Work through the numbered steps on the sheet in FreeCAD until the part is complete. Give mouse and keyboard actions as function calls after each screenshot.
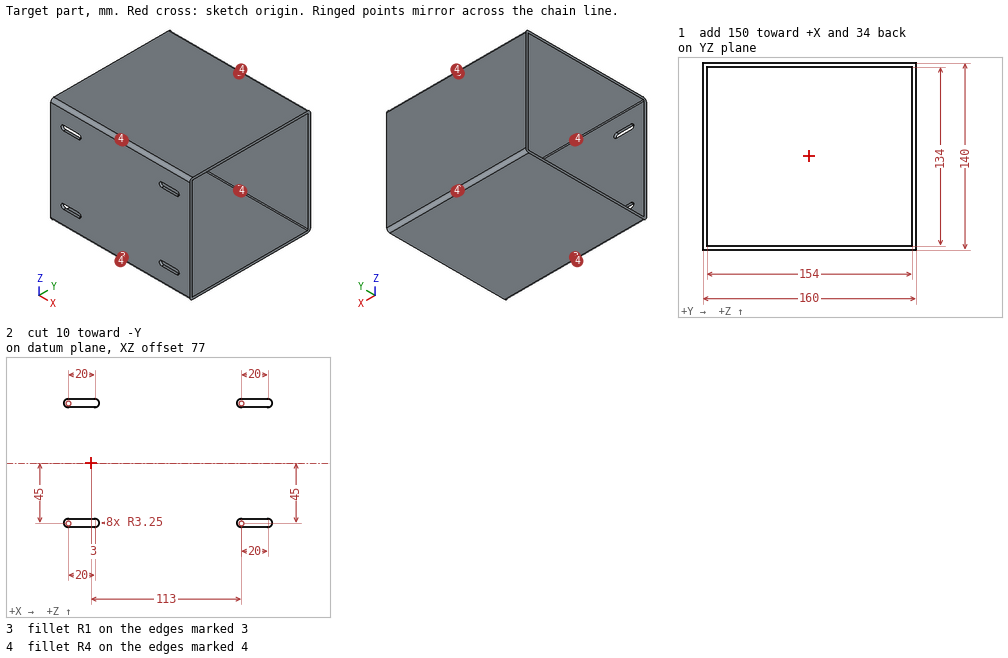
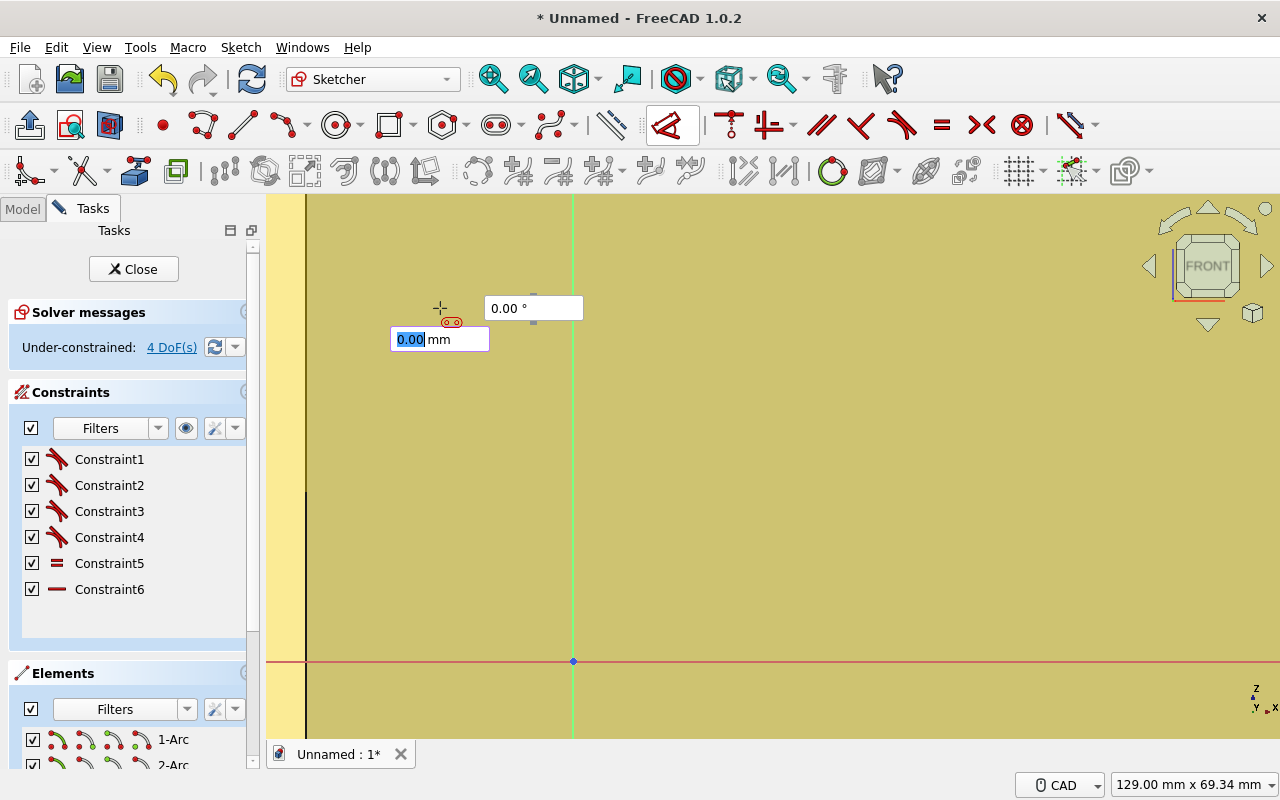
click(597, 308)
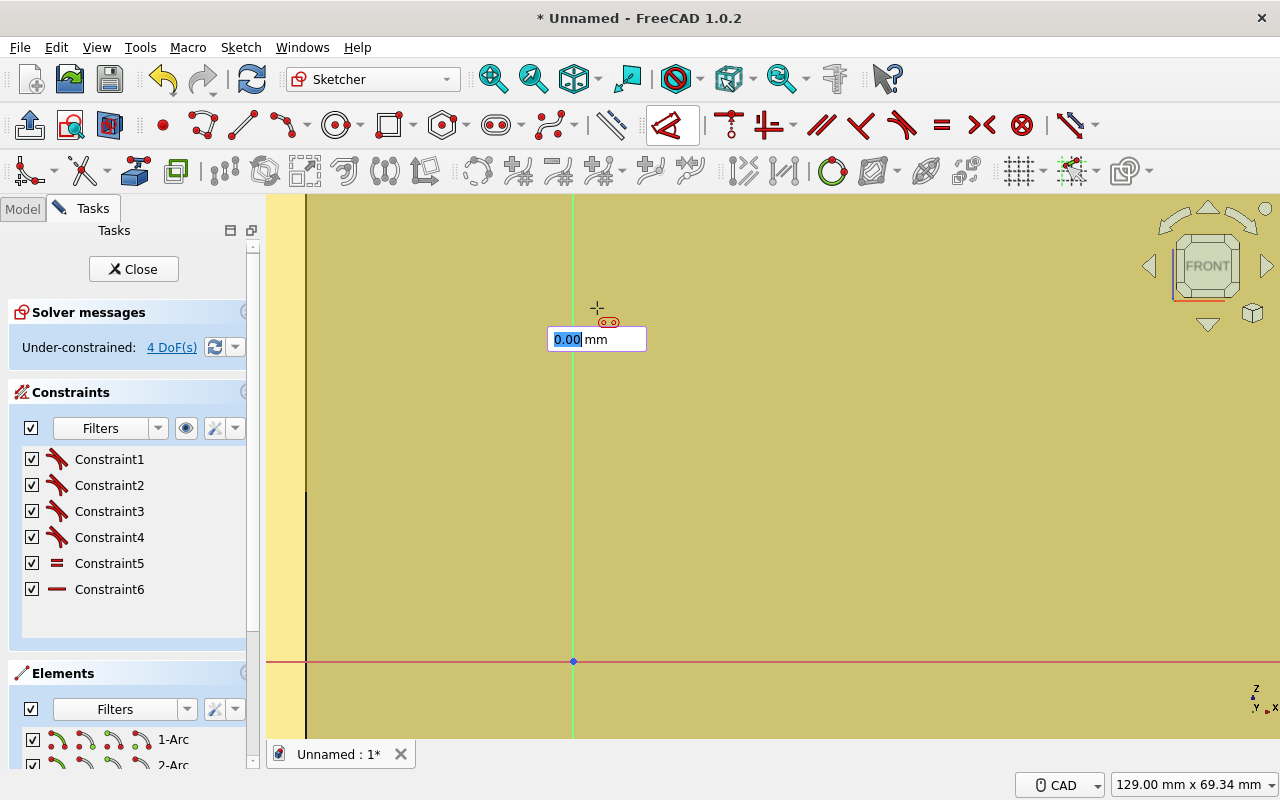
click(518, 282)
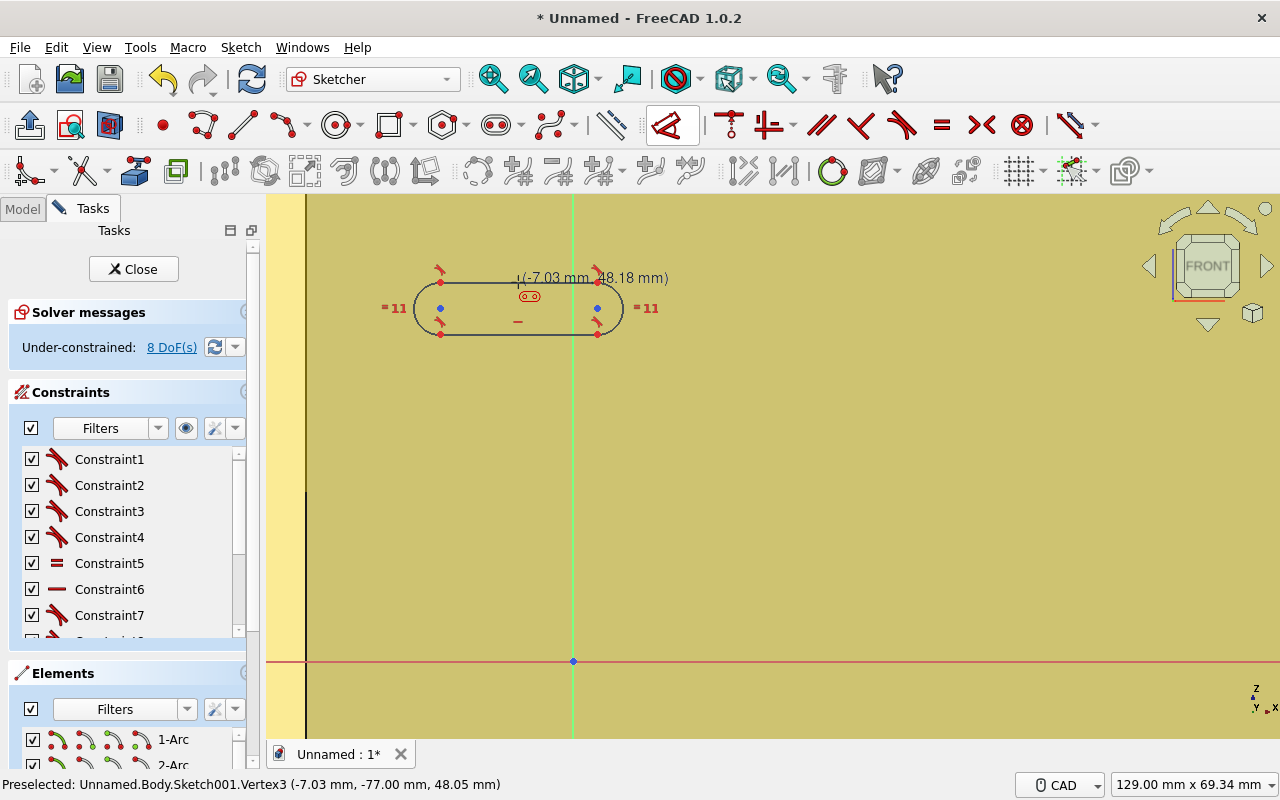
scroll(440, 307, down, 4)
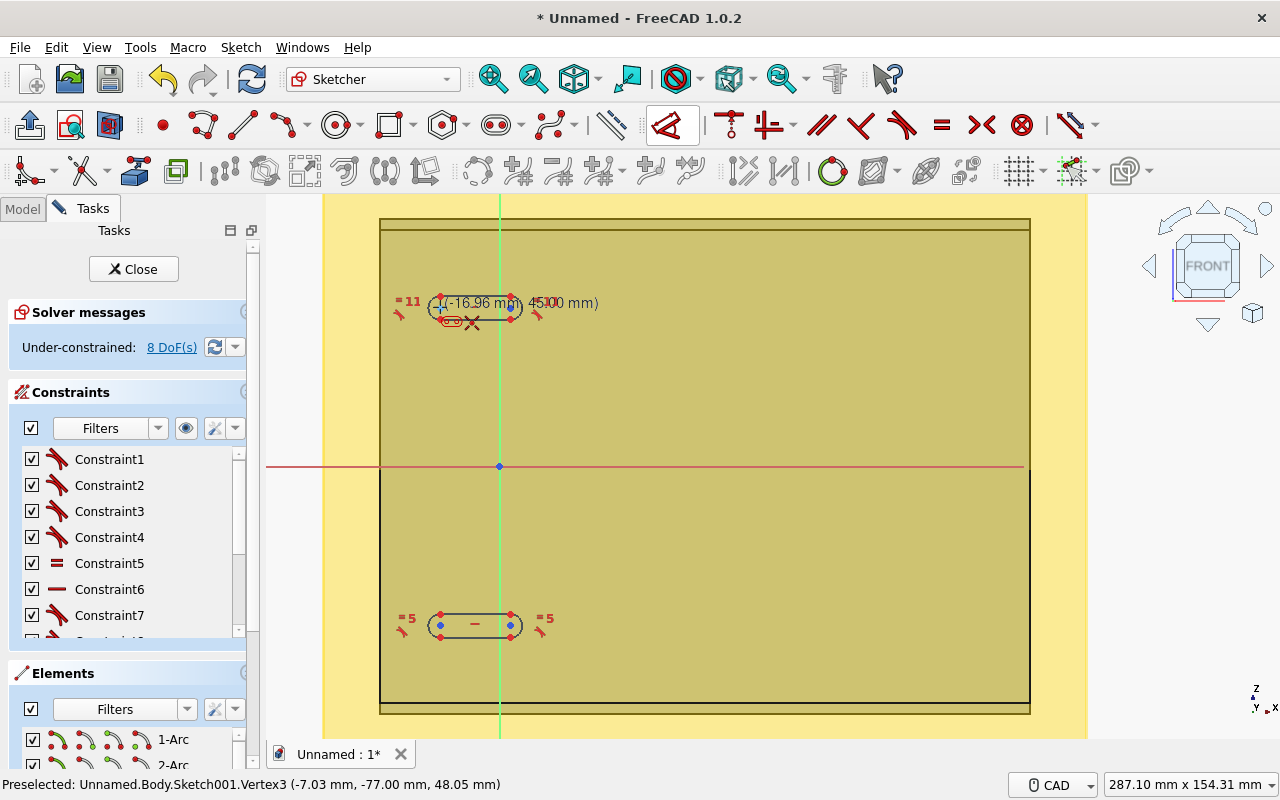
scroll(899, 625, up, 4)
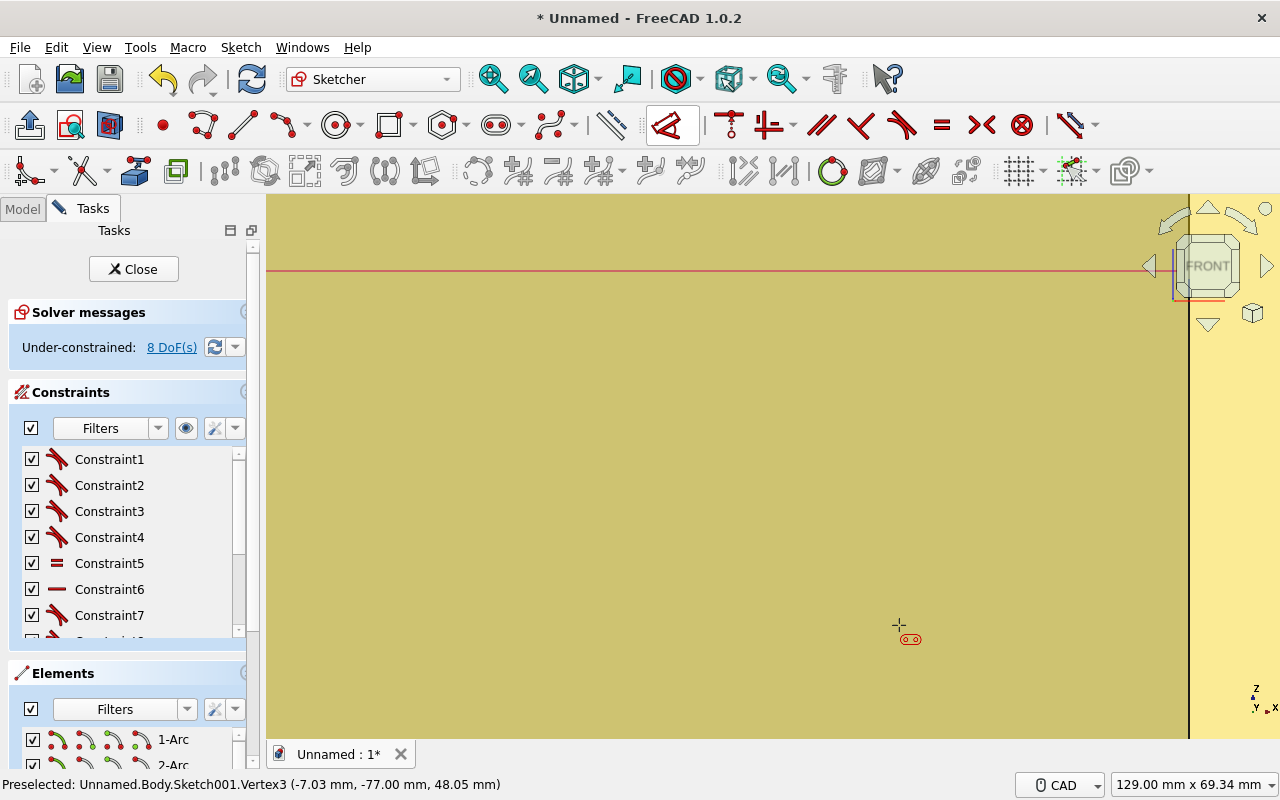
click(898, 625)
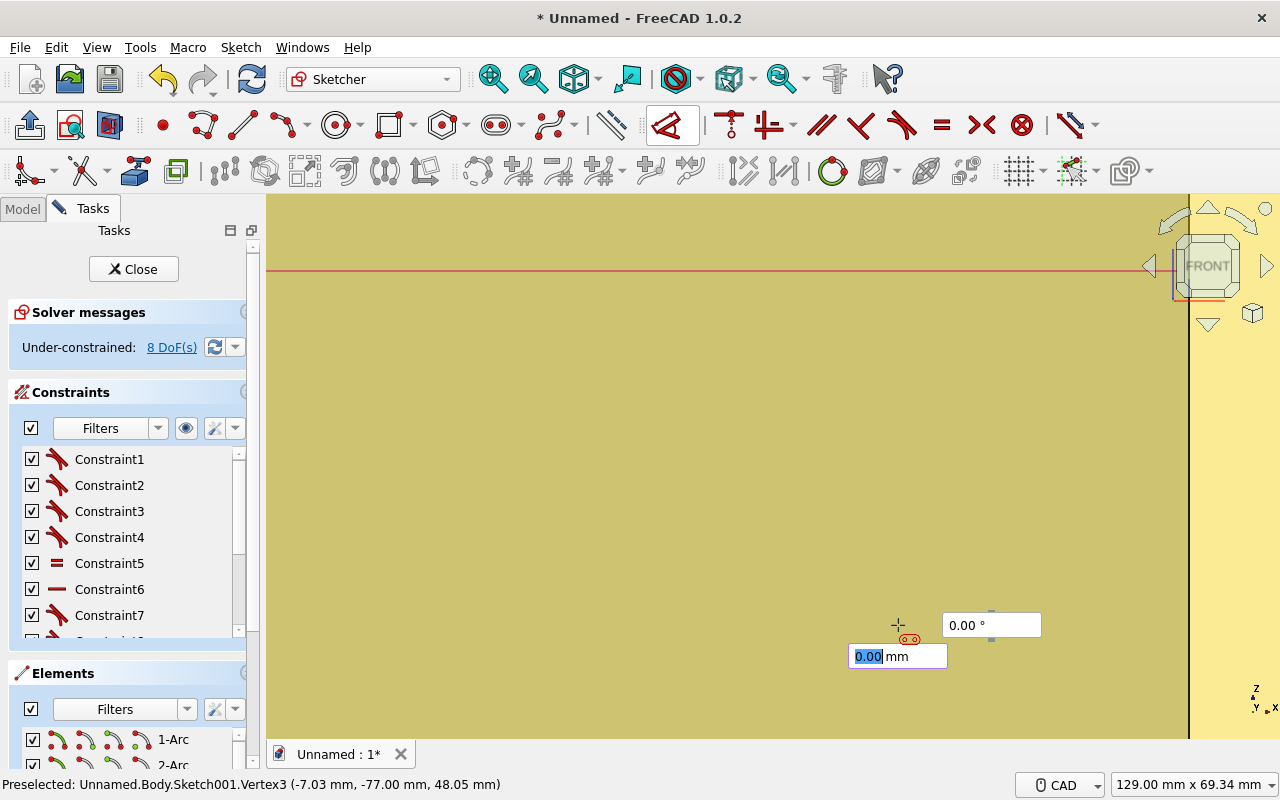
click(1056, 625)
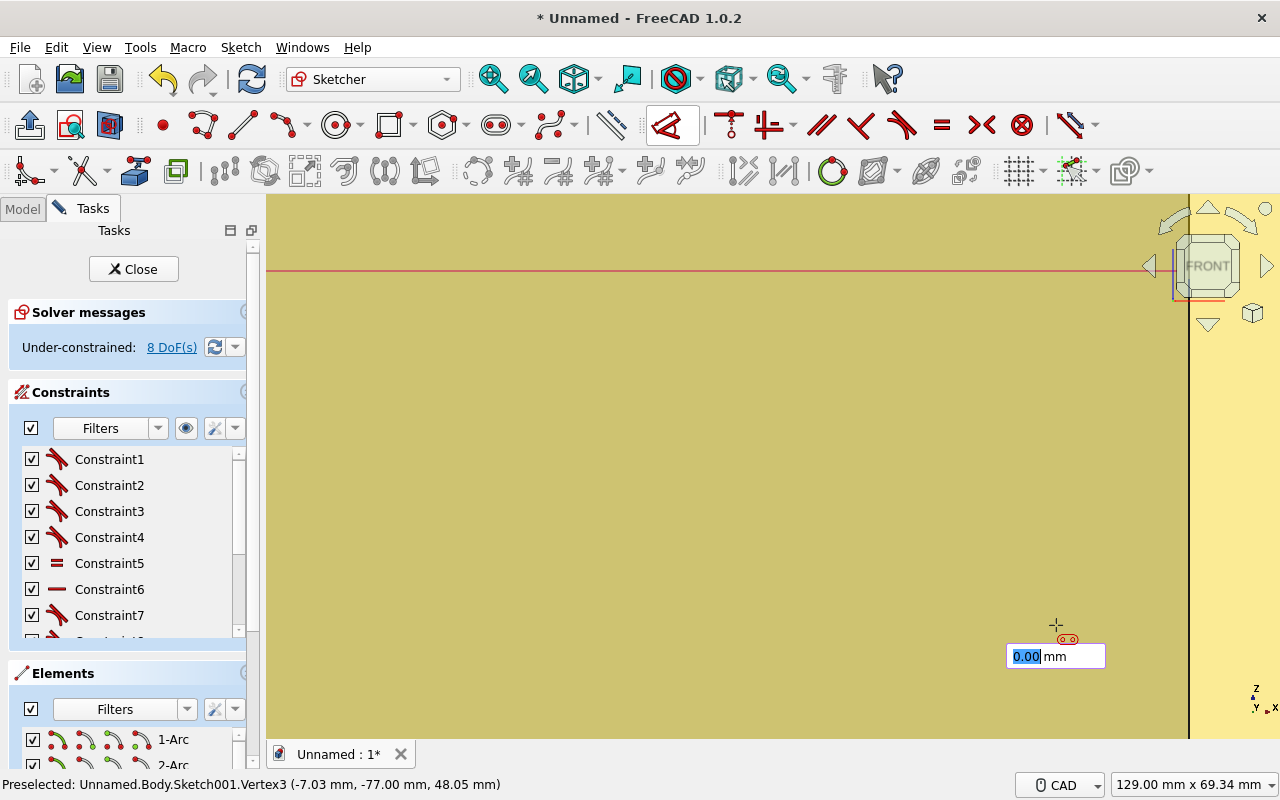
click(977, 651)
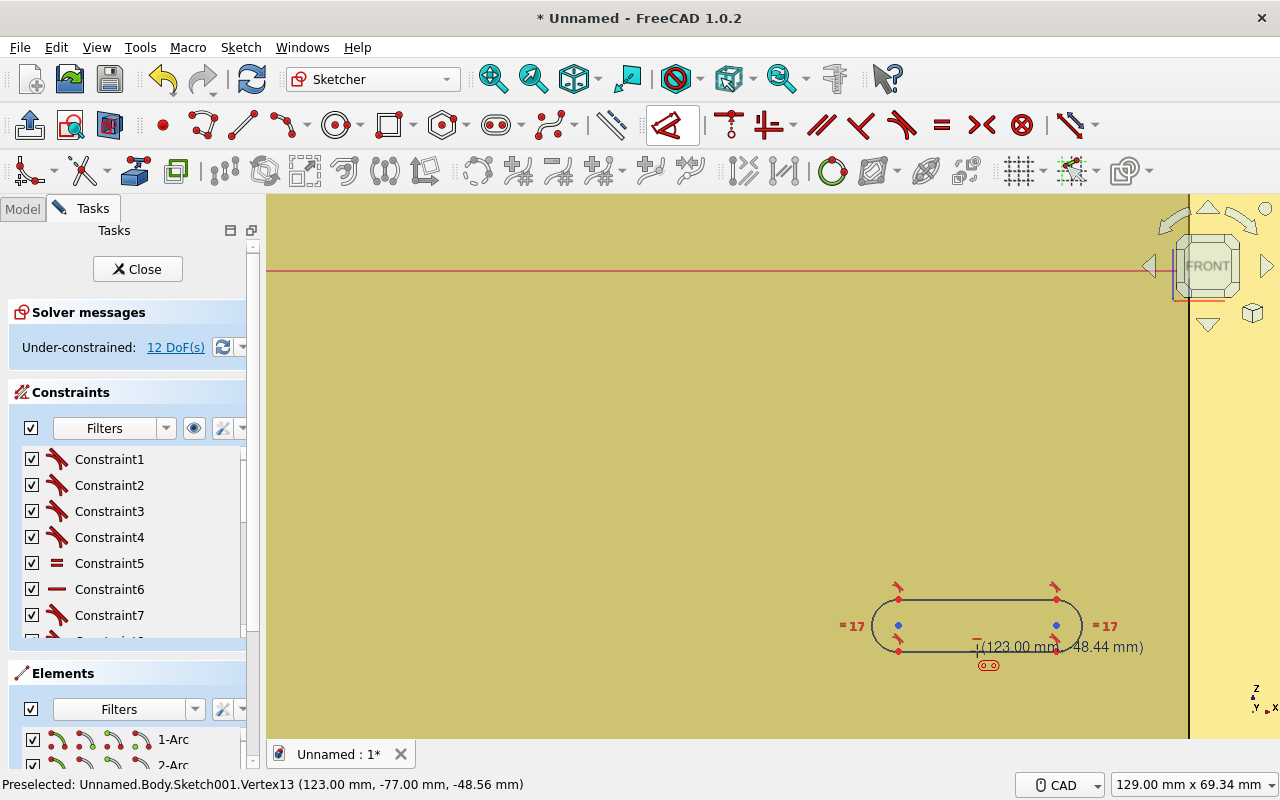
scroll(899, 626, down, 4)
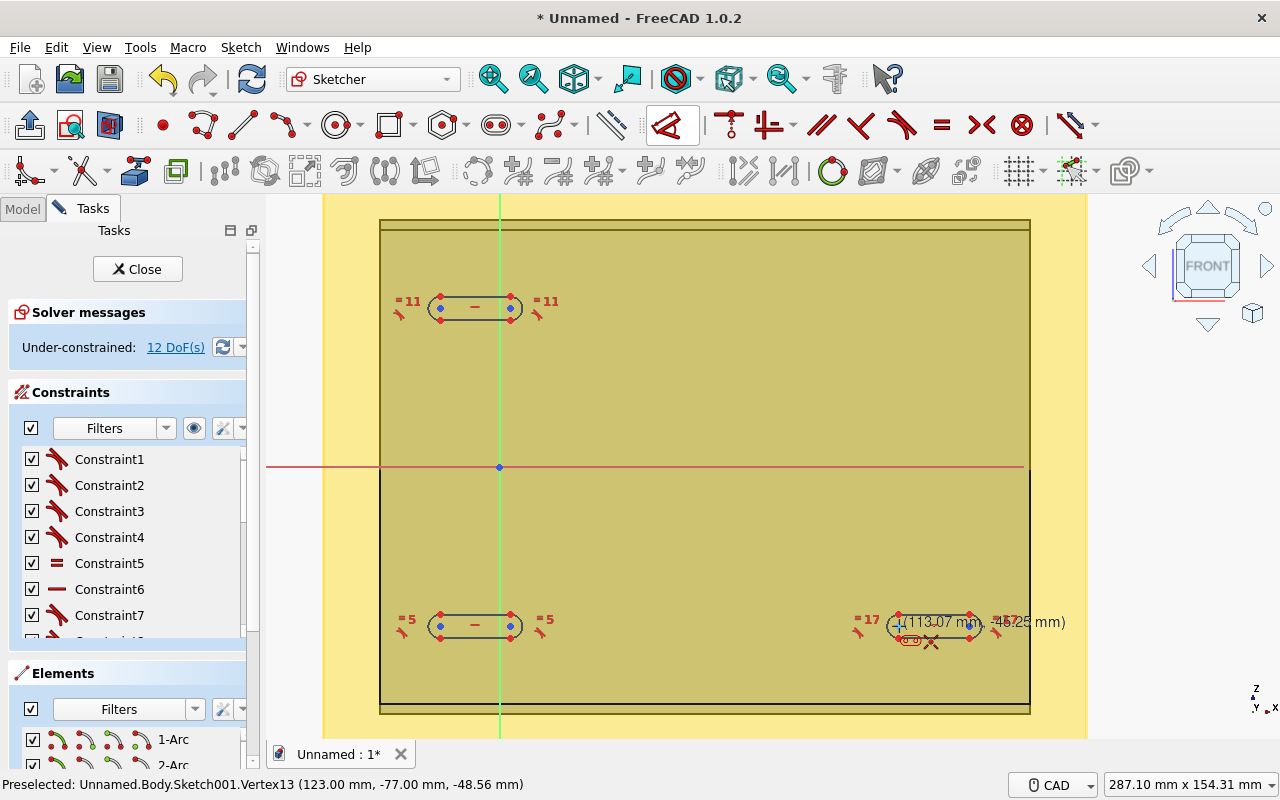
scroll(899, 308, up, 4)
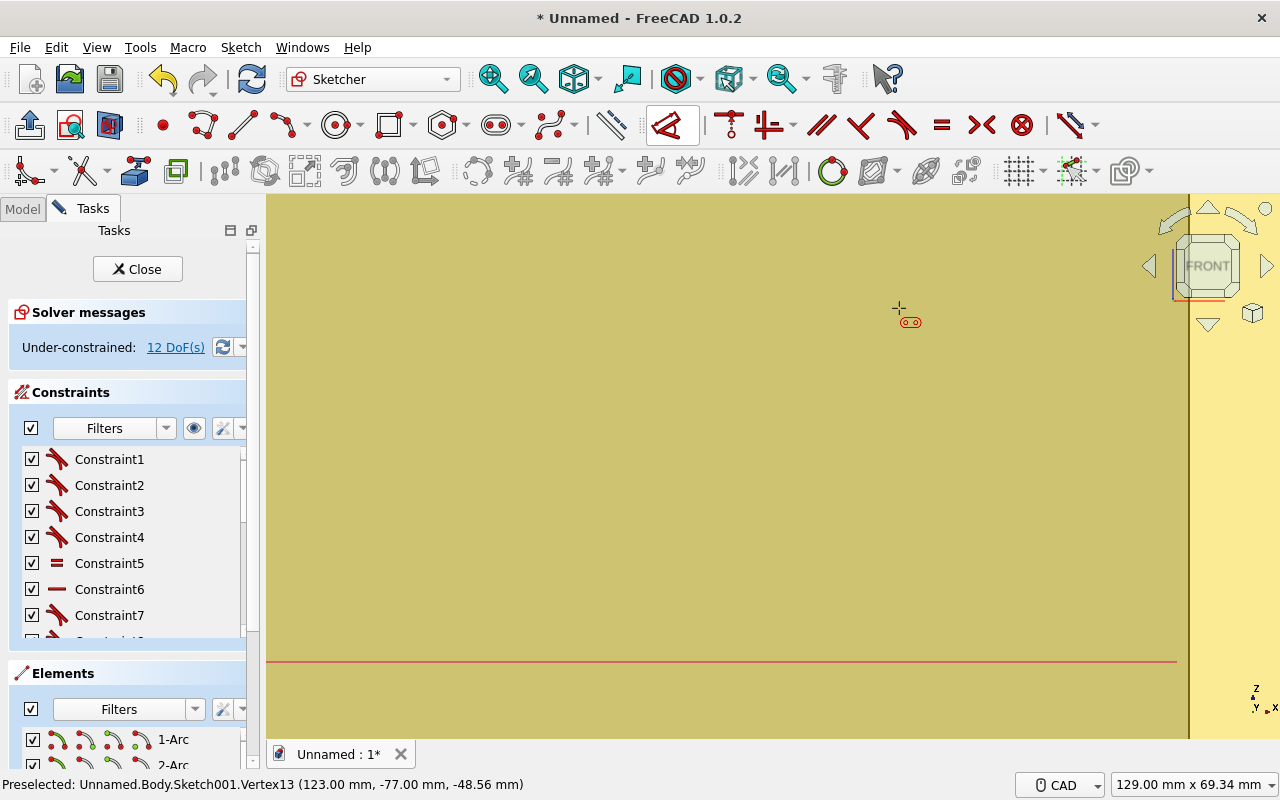
click(898, 308)